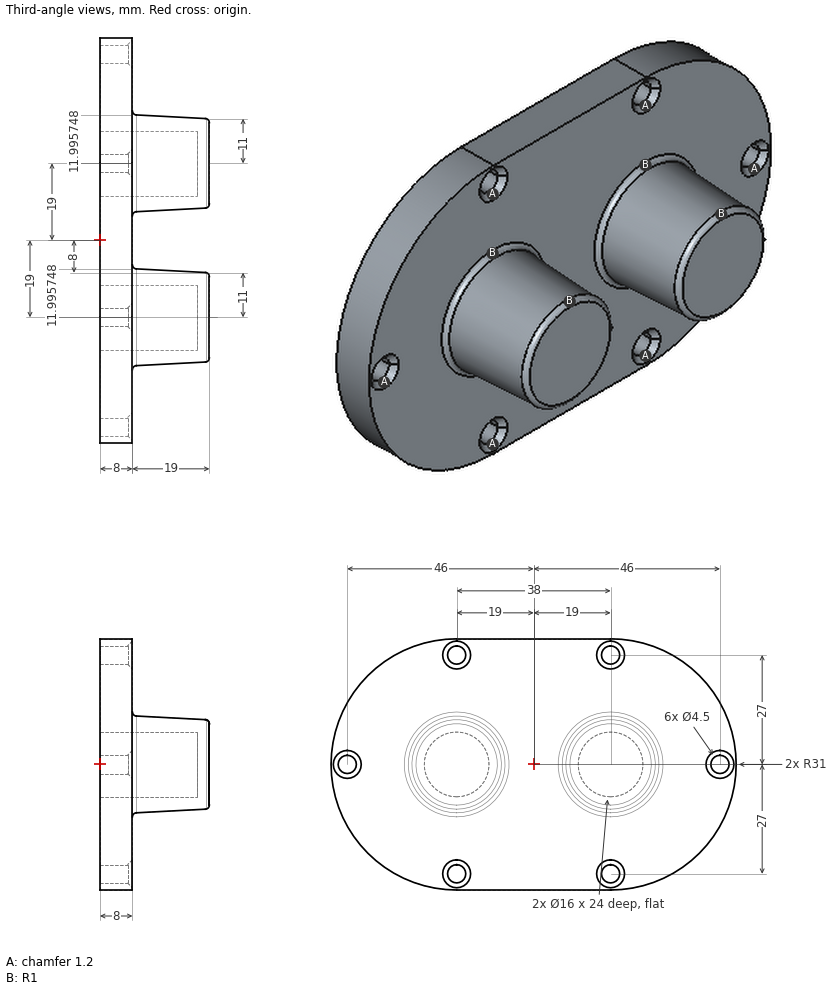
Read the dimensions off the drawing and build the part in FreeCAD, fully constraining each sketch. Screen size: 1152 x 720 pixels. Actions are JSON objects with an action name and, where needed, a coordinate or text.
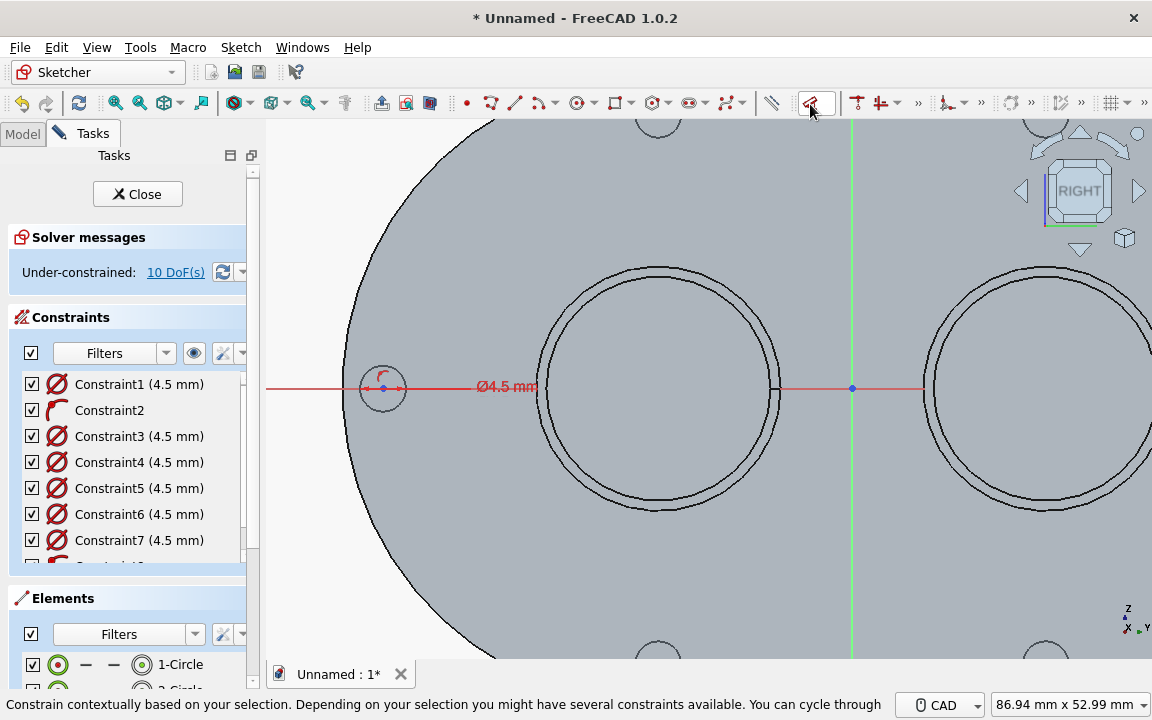
{"action": "scroll", "coordinate": [383, 389], "scroll_direction": "down", "scroll_amount": 3}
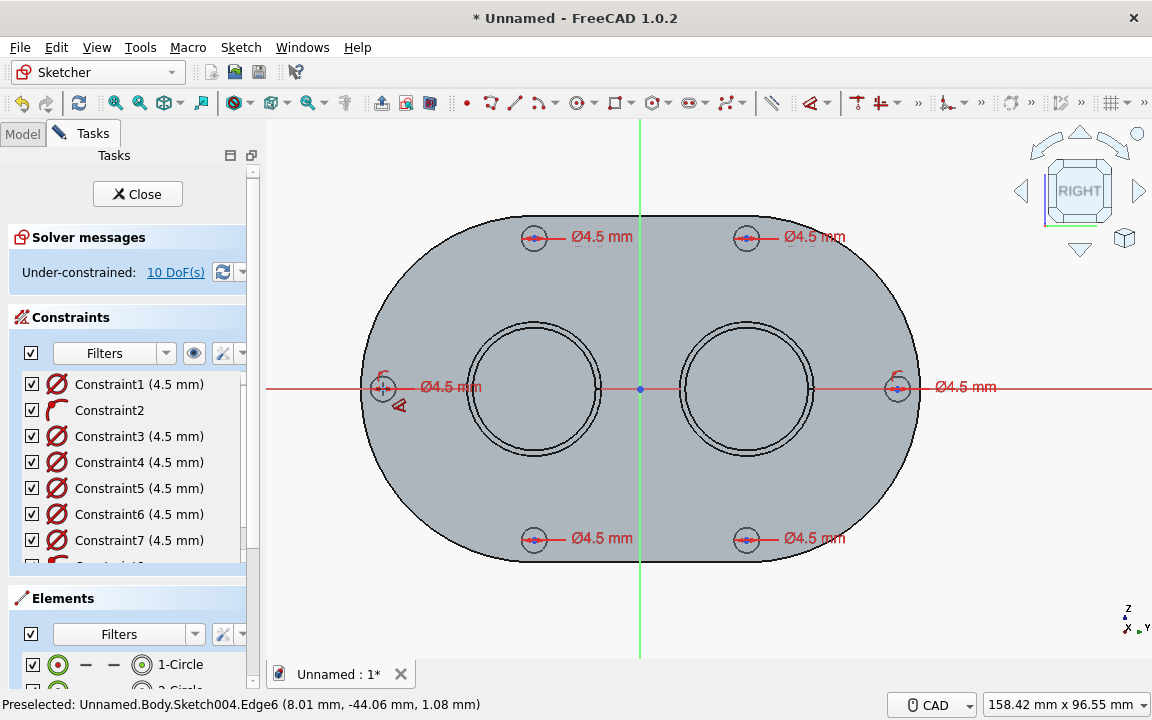
{"action": "left_click", "coordinate": [898, 389]}
{"action": "left_click", "coordinate": [769, 423]}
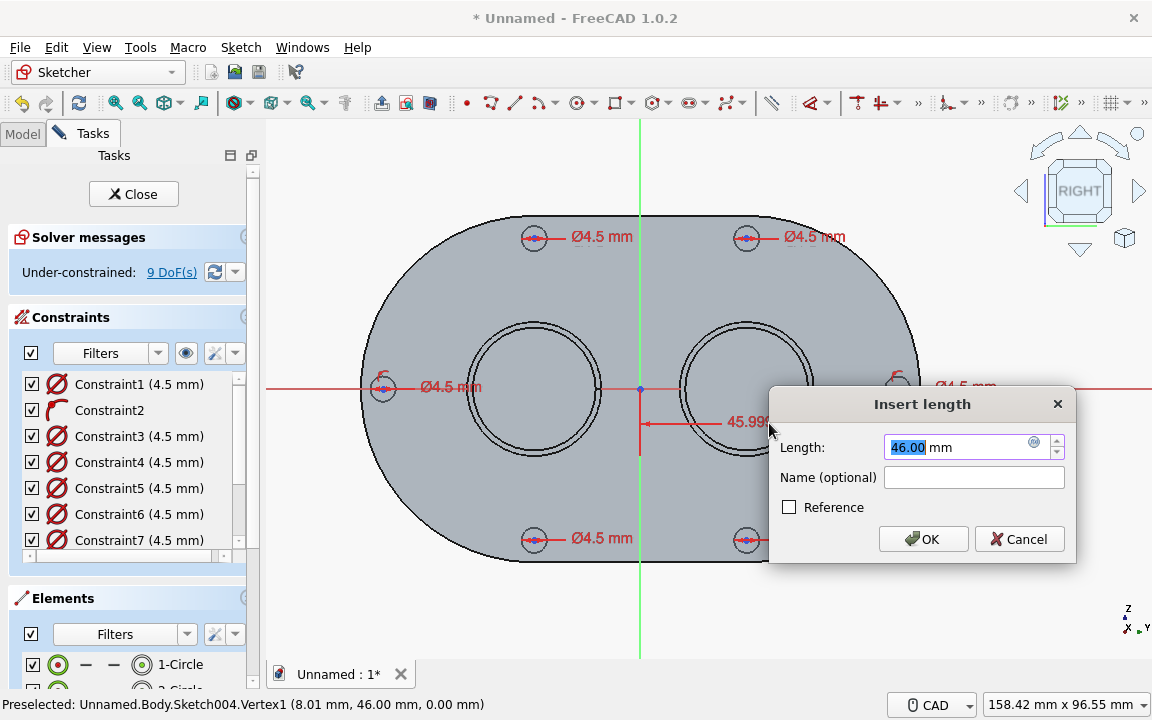
{"action": "type", "text": "46"}
{"action": "key", "text": "Return"}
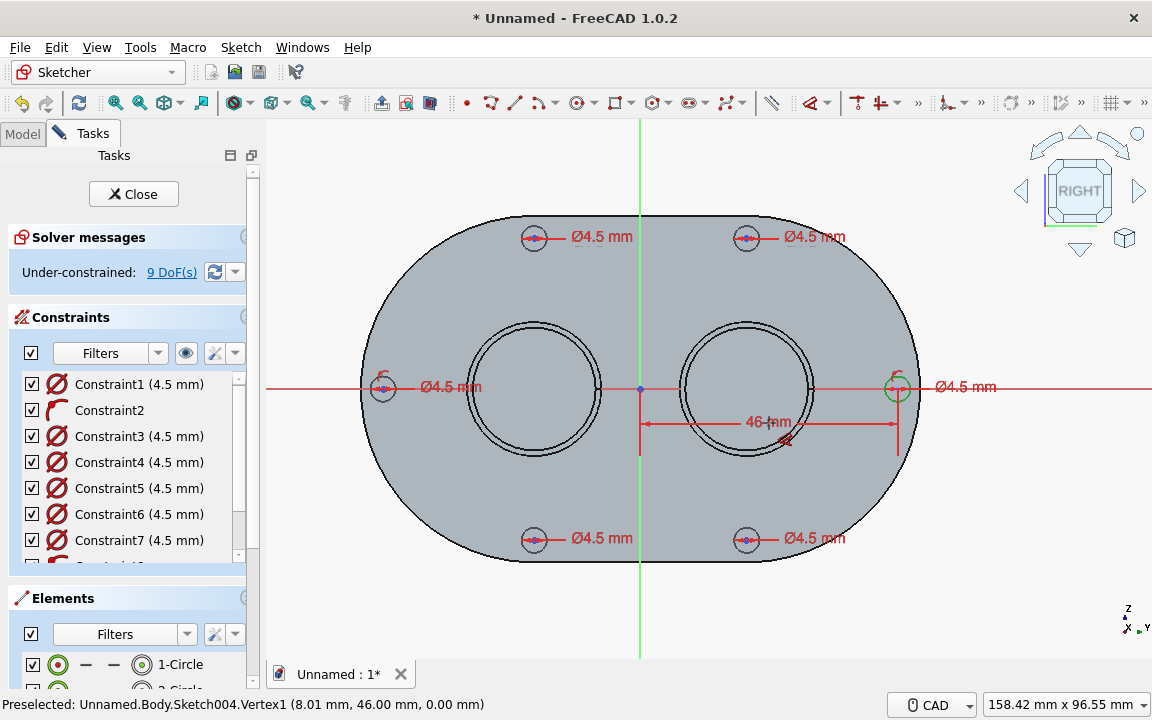
{"action": "left_click", "coordinate": [747, 239]}
{"action": "left_click", "coordinate": [694, 205]}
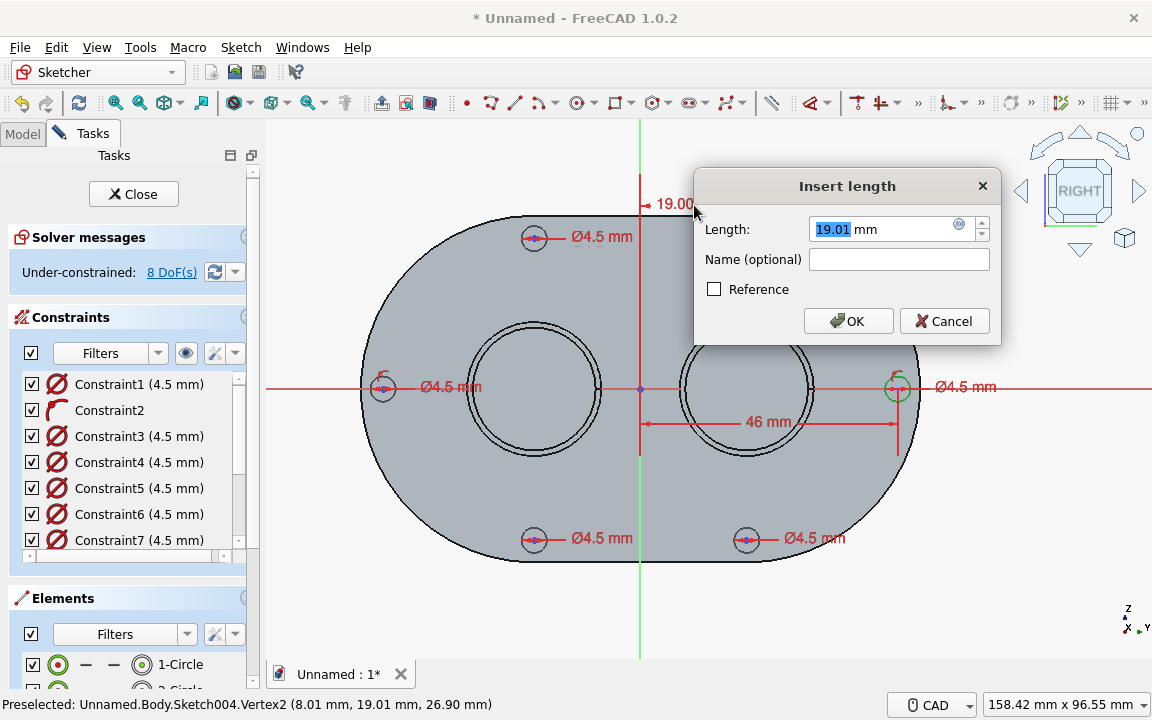
{"action": "type", "text": "19"}
{"action": "key", "text": "Return"}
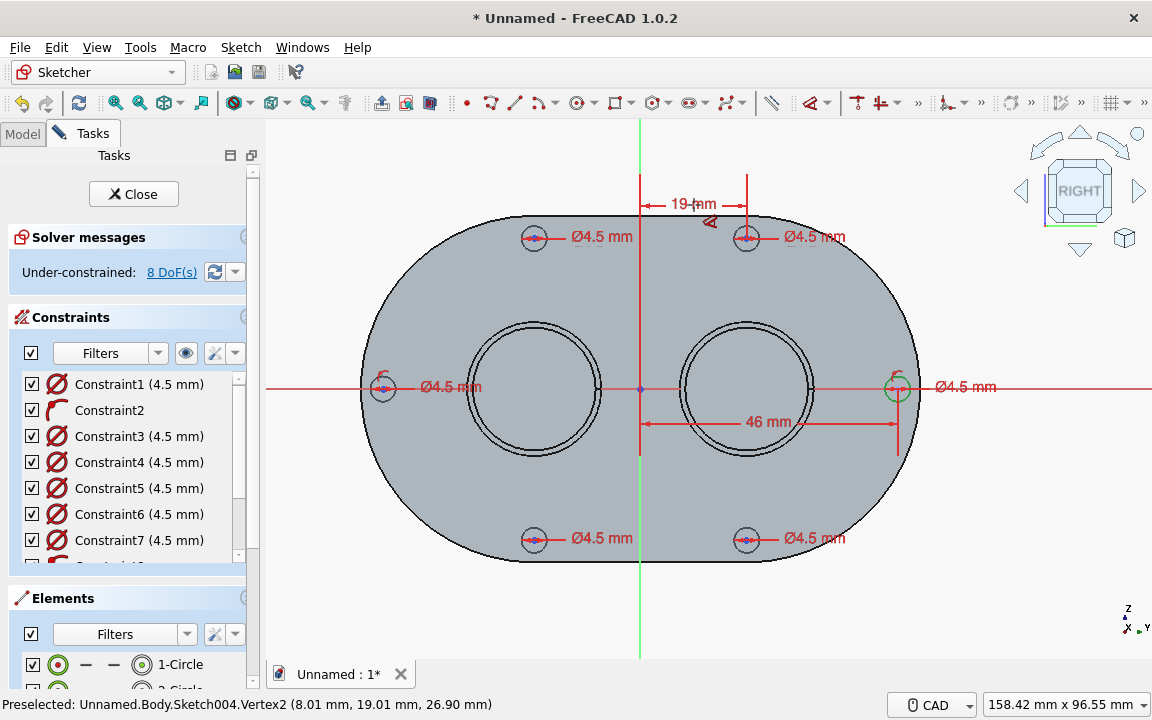
{"action": "left_click", "coordinate": [747, 239]}
{"action": "left_click", "coordinate": [781, 314]}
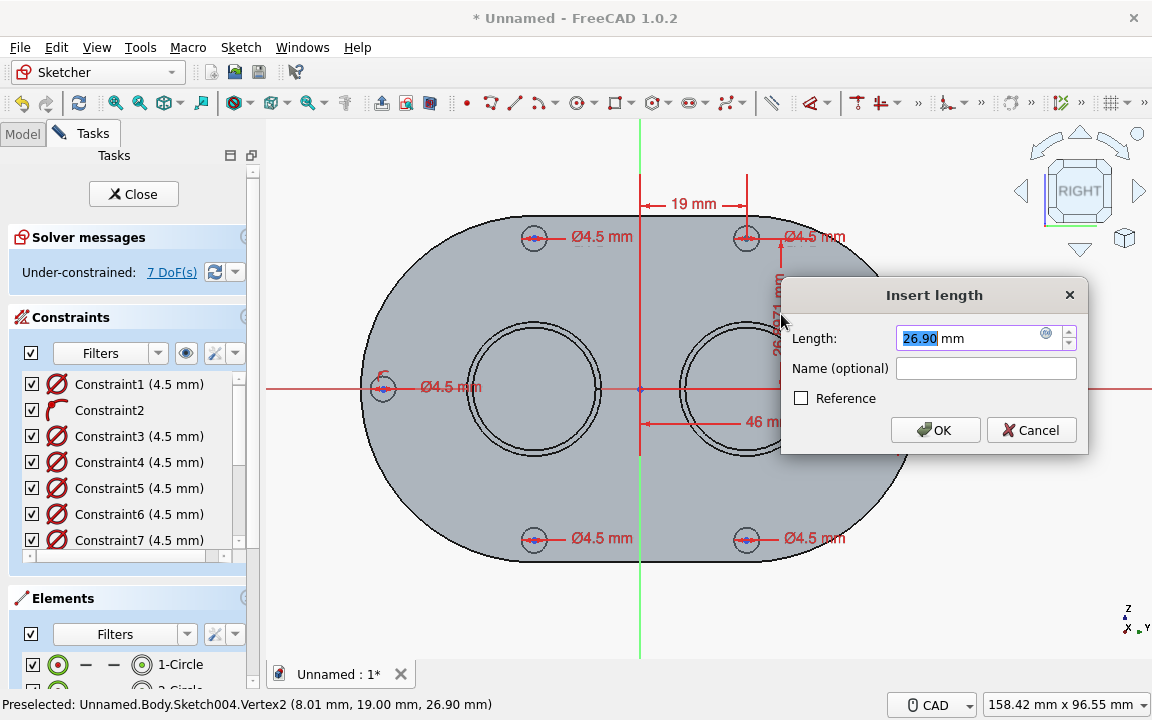
{"action": "type", "text": "27"}
{"action": "key", "text": "Return"}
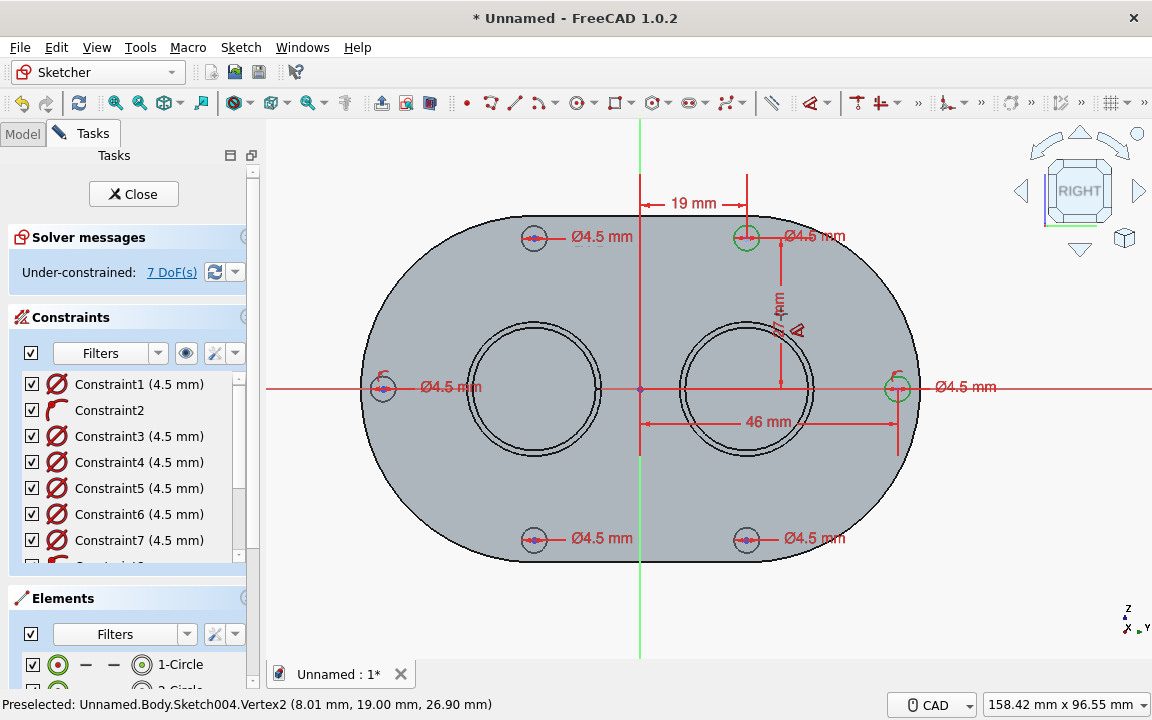
{"action": "left_click", "coordinate": [747, 540]}
{"action": "left_click", "coordinate": [694, 574]}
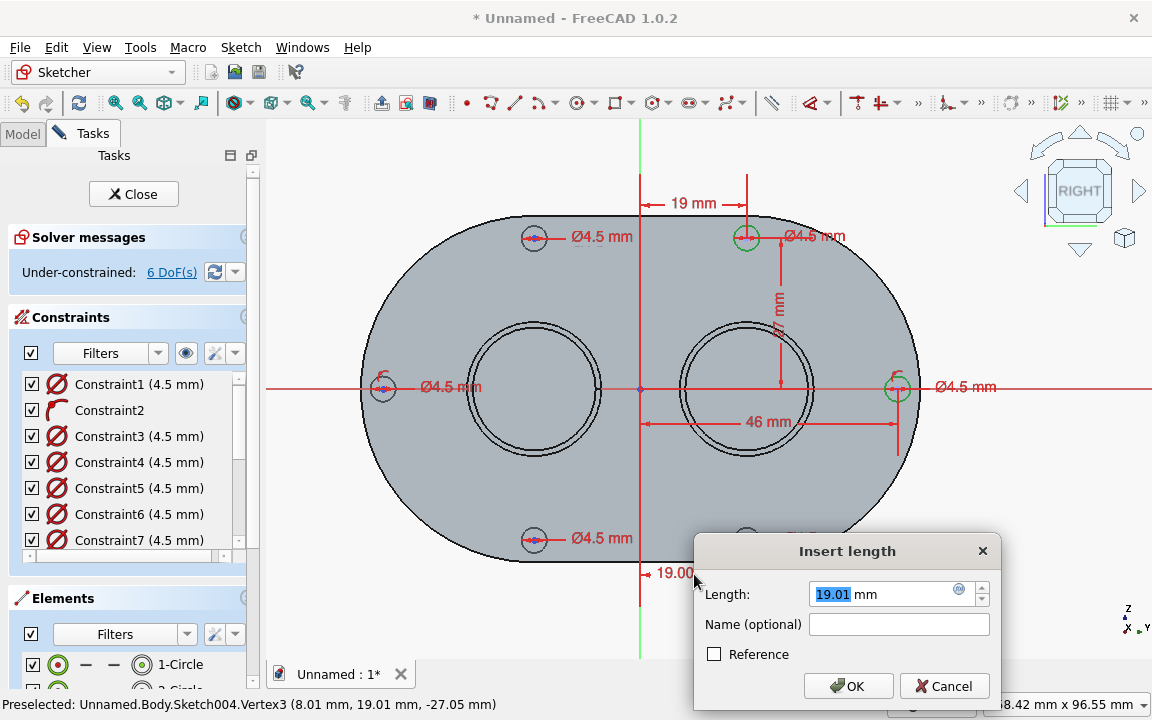
{"action": "type", "text": "19"}
{"action": "key", "text": "Return"}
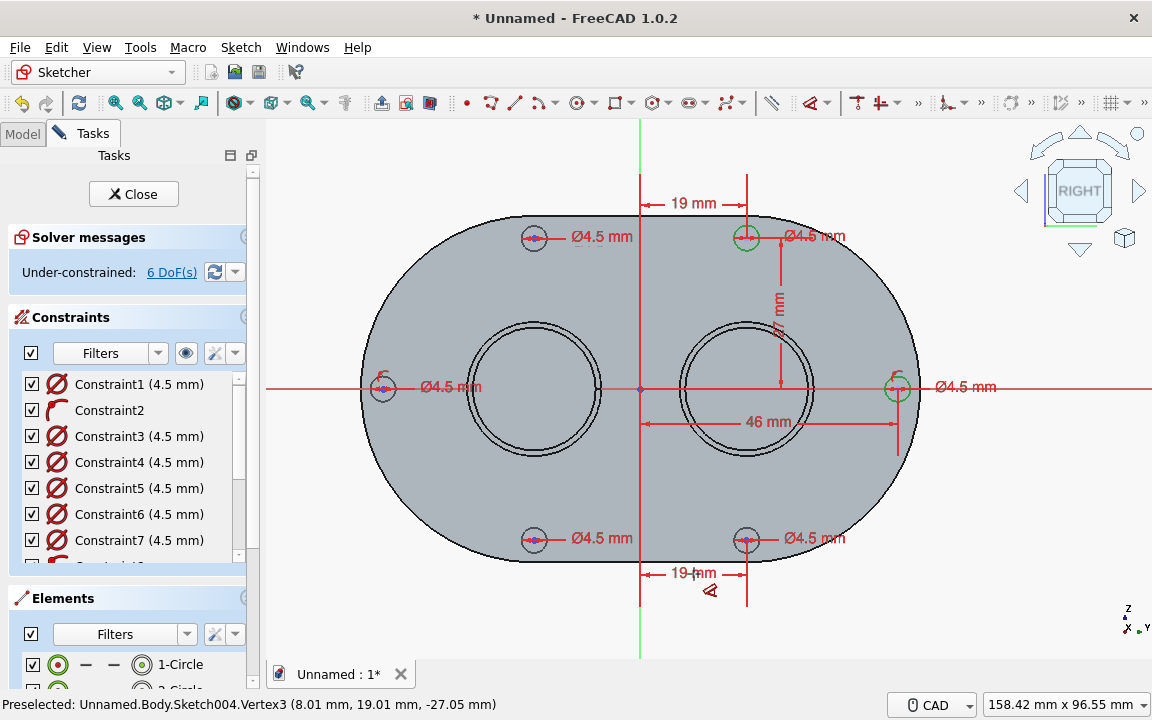
{"action": "left_click", "coordinate": [747, 540]}
{"action": "left_click", "coordinate": [781, 465]}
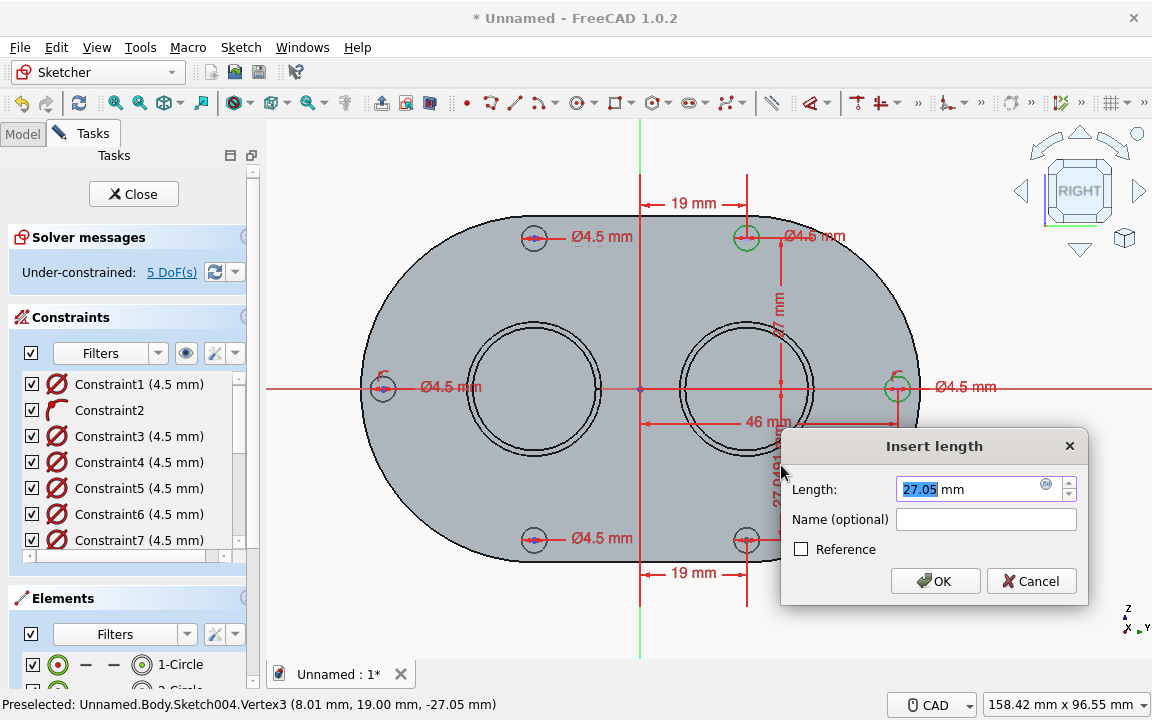
{"action": "type", "text": "27"}
{"action": "key", "text": "Return"}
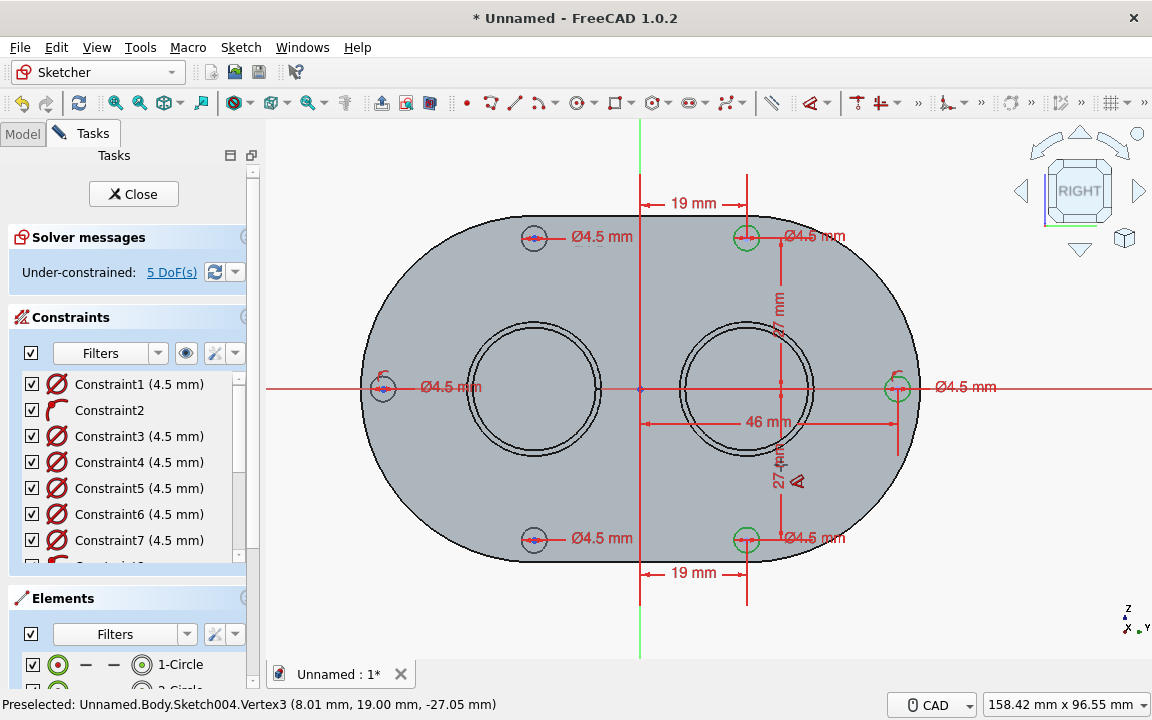
{"action": "left_click", "coordinate": [534, 239]}
{"action": "left_click", "coordinate": [587, 205]}